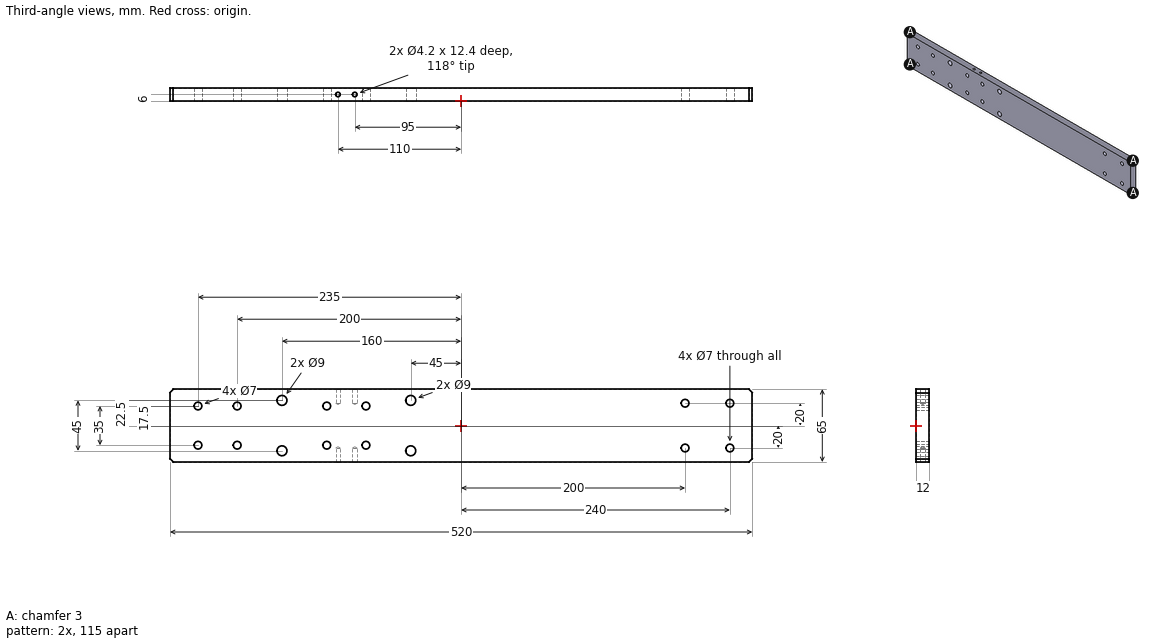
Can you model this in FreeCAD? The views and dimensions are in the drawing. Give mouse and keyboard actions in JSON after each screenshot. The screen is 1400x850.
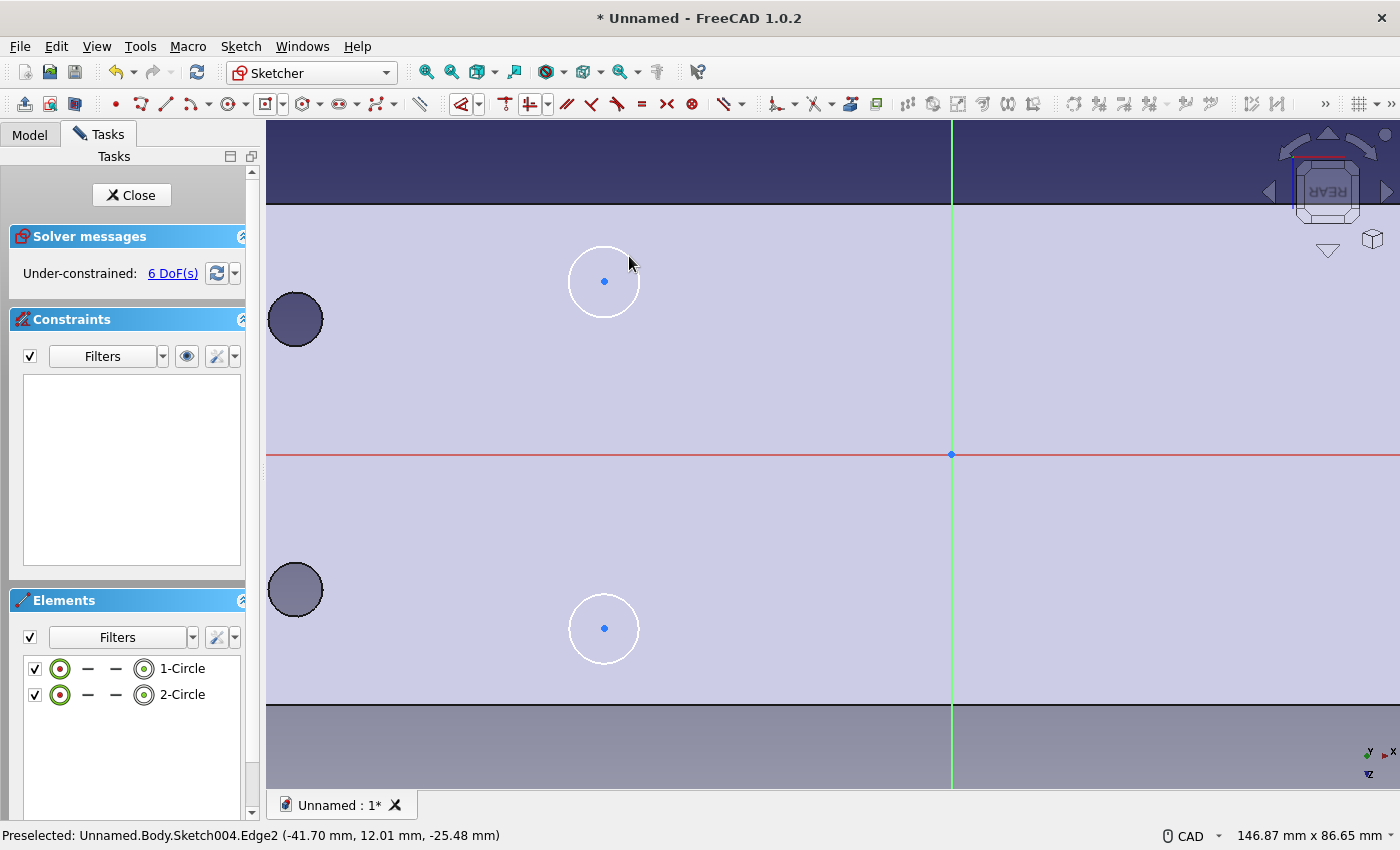
{"action": "left_click", "coordinate": [628, 604]}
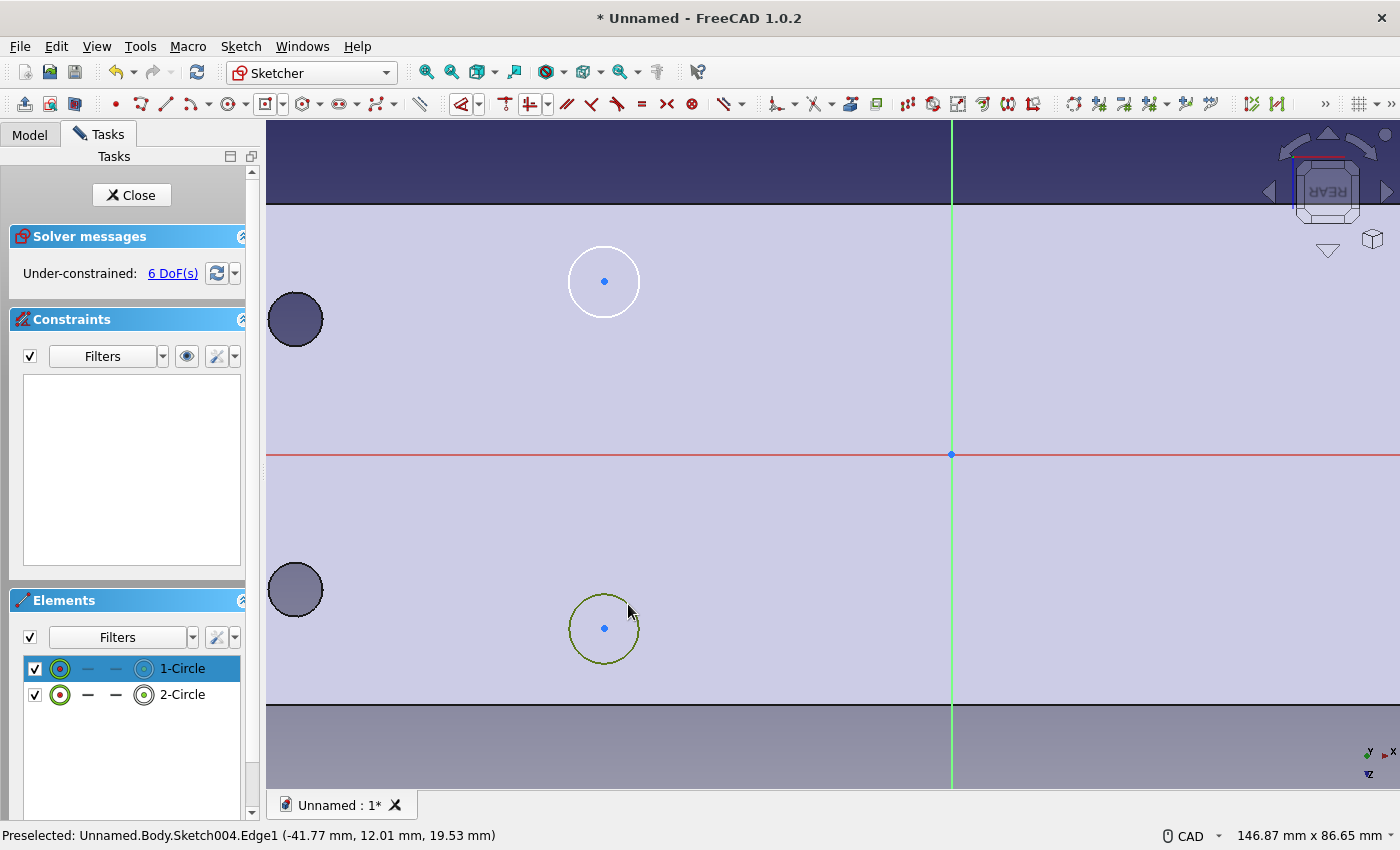
{"action": "left_click", "coordinate": [629, 257]}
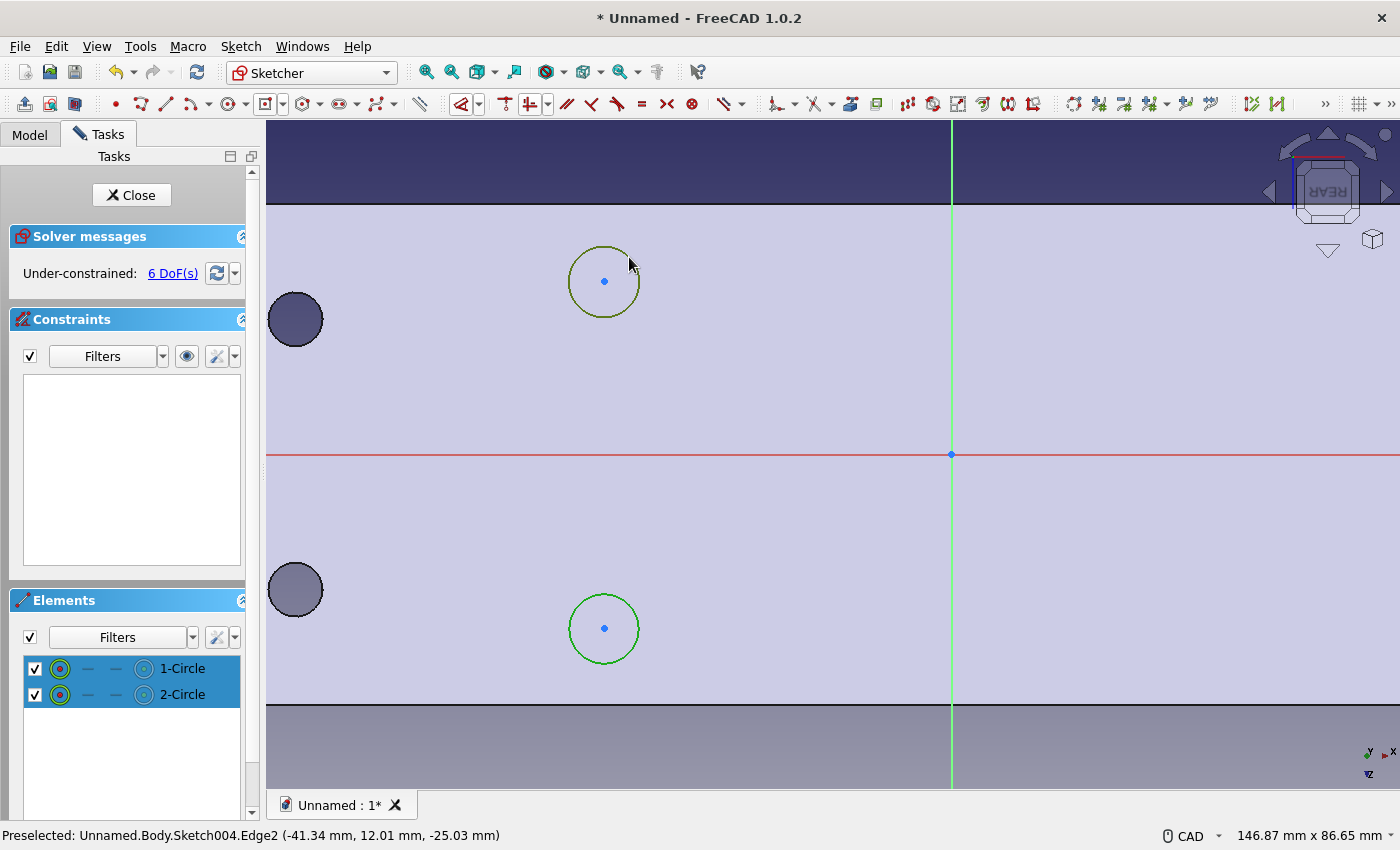
{"action": "left_click", "coordinate": [642, 104]}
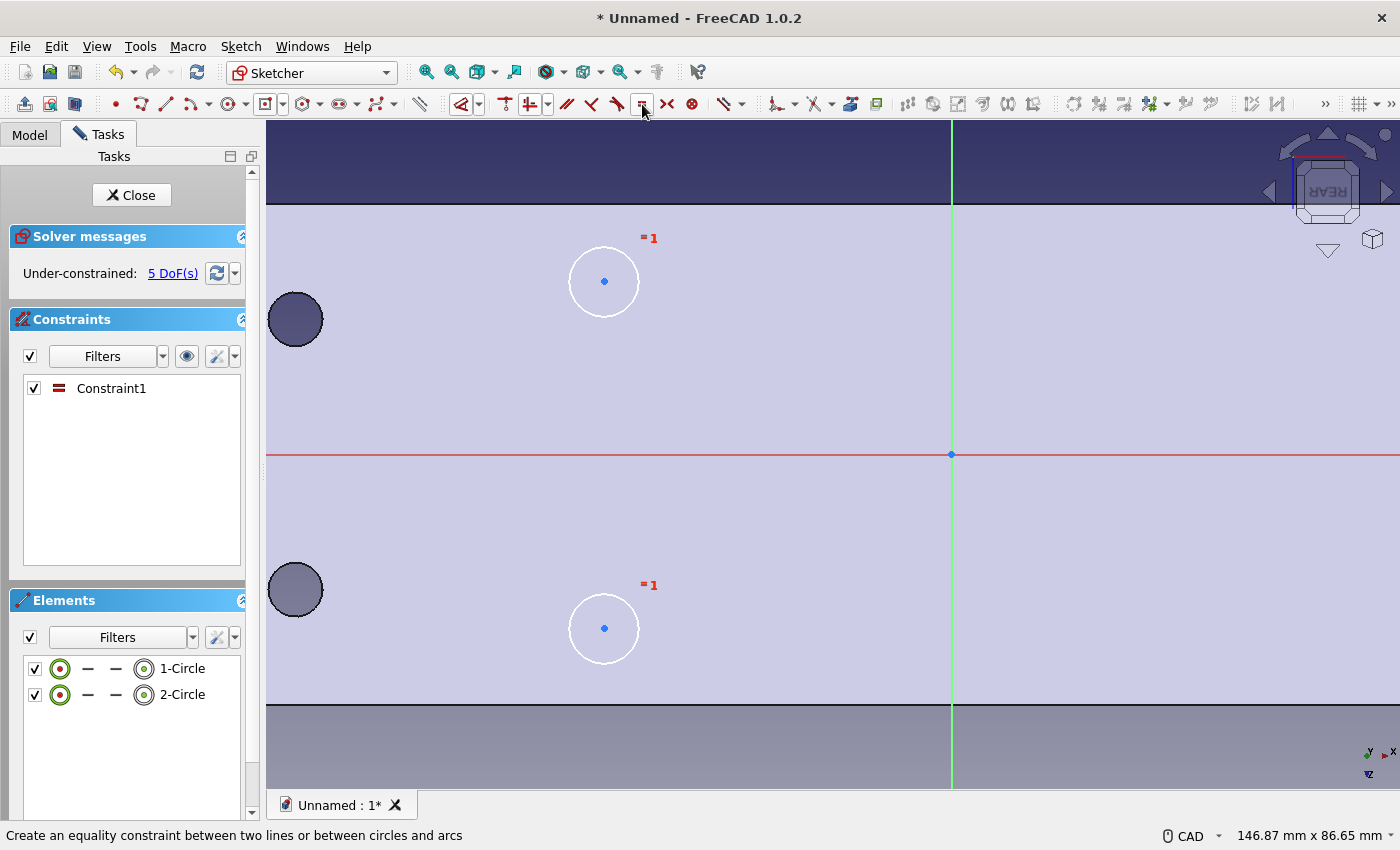
{"action": "left_click", "coordinate": [604, 629]}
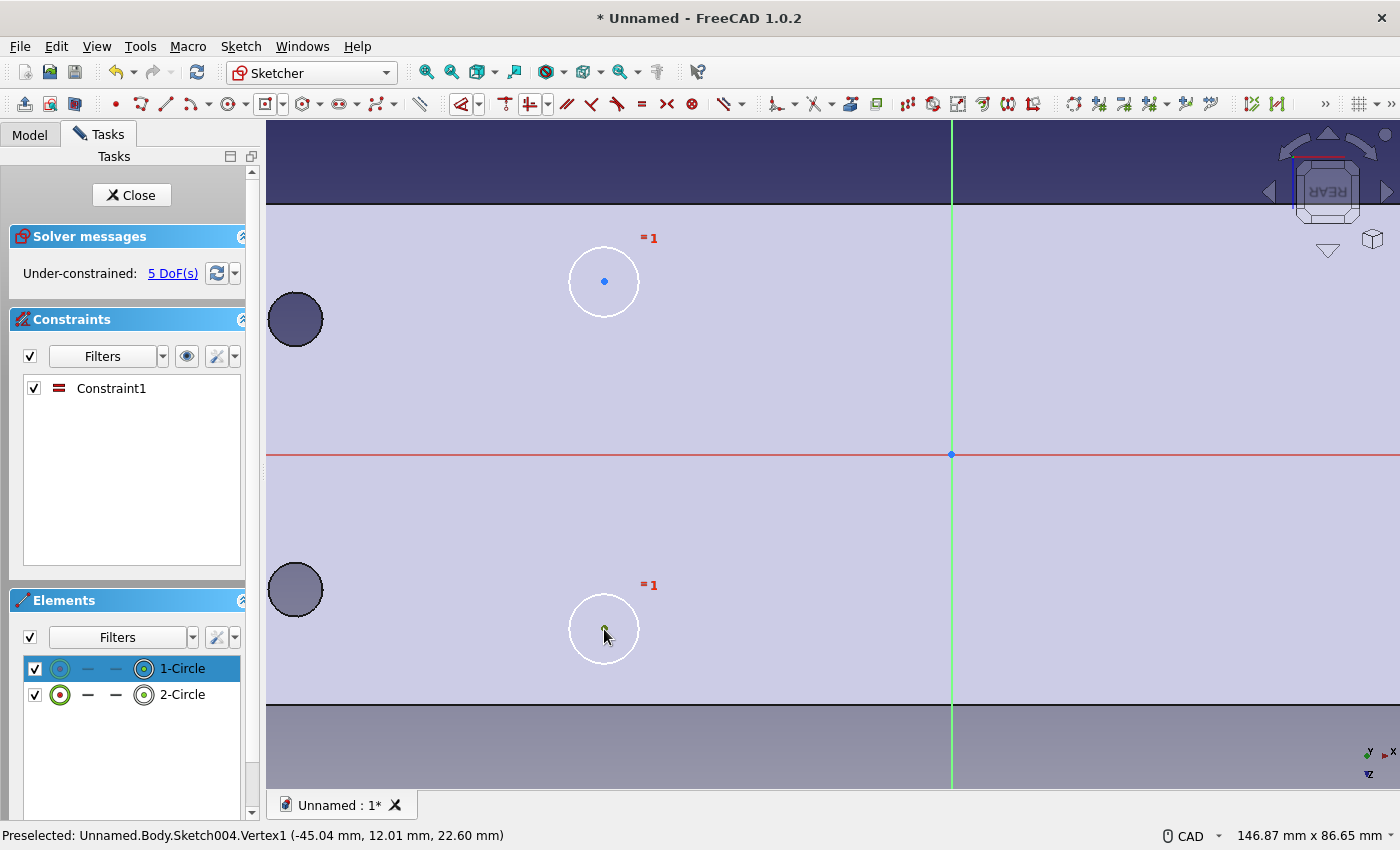
{"action": "left_click", "coordinate": [604, 282]}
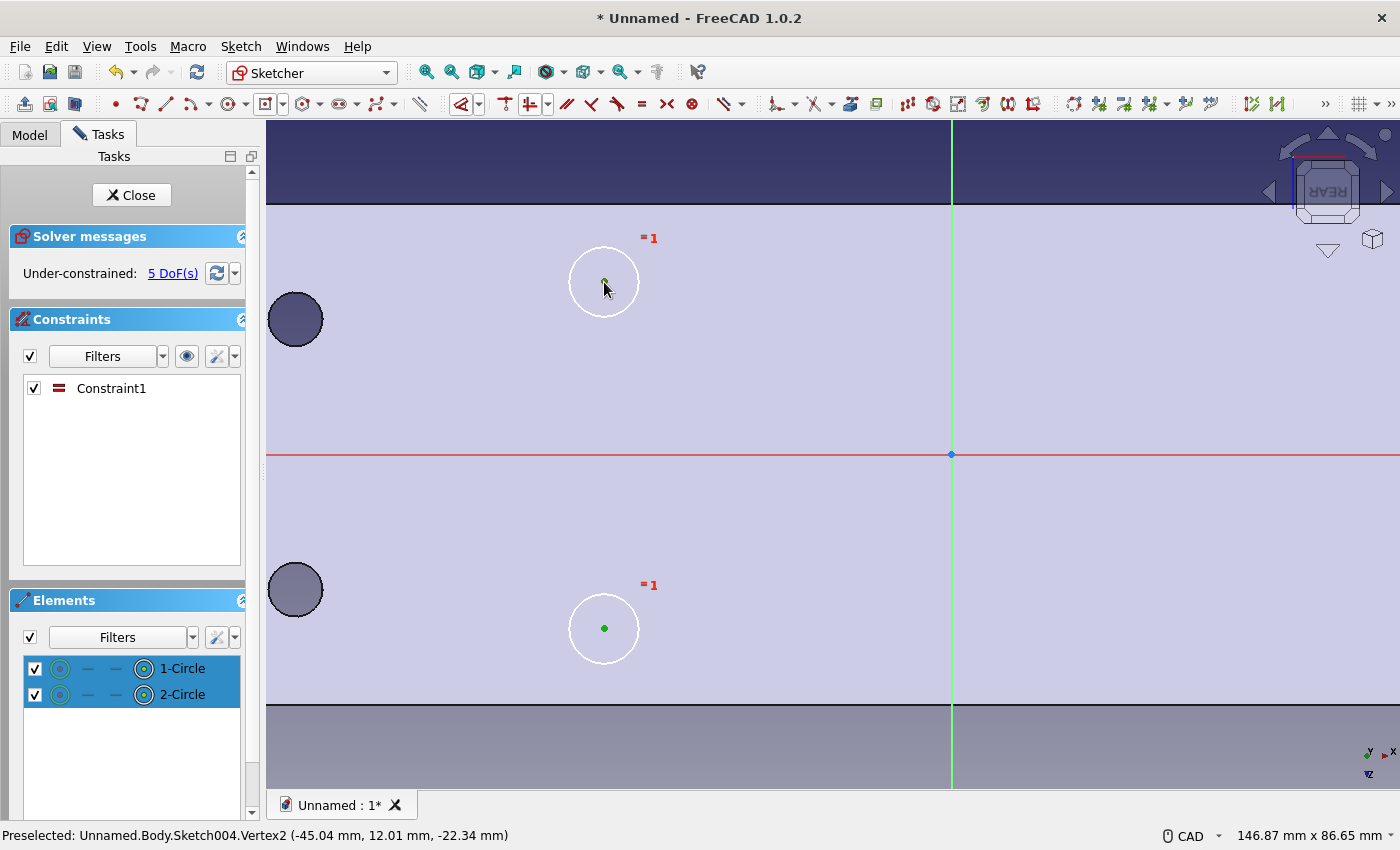
{"action": "left_click", "coordinate": [548, 104]}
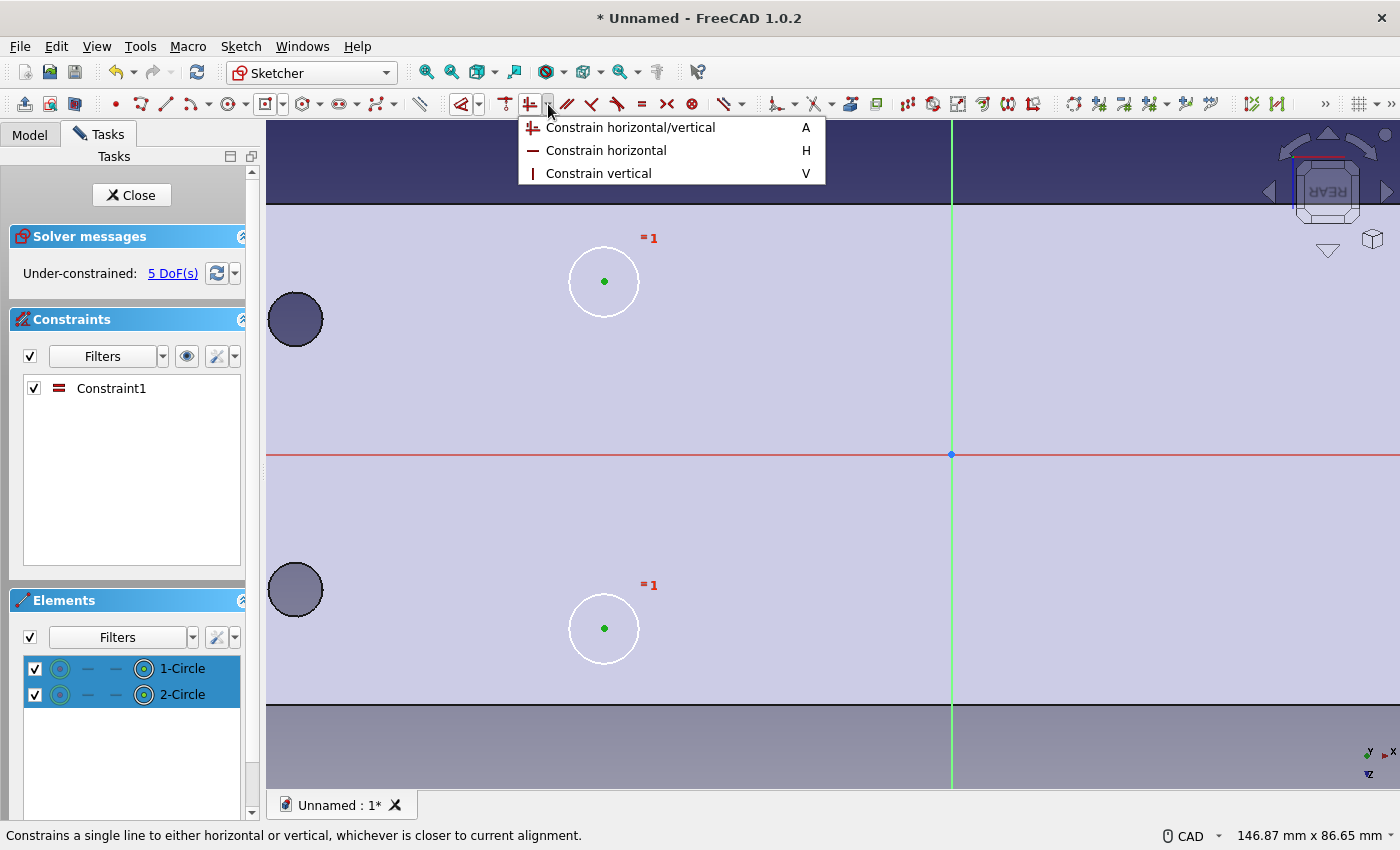
{"action": "left_click", "coordinate": [672, 174]}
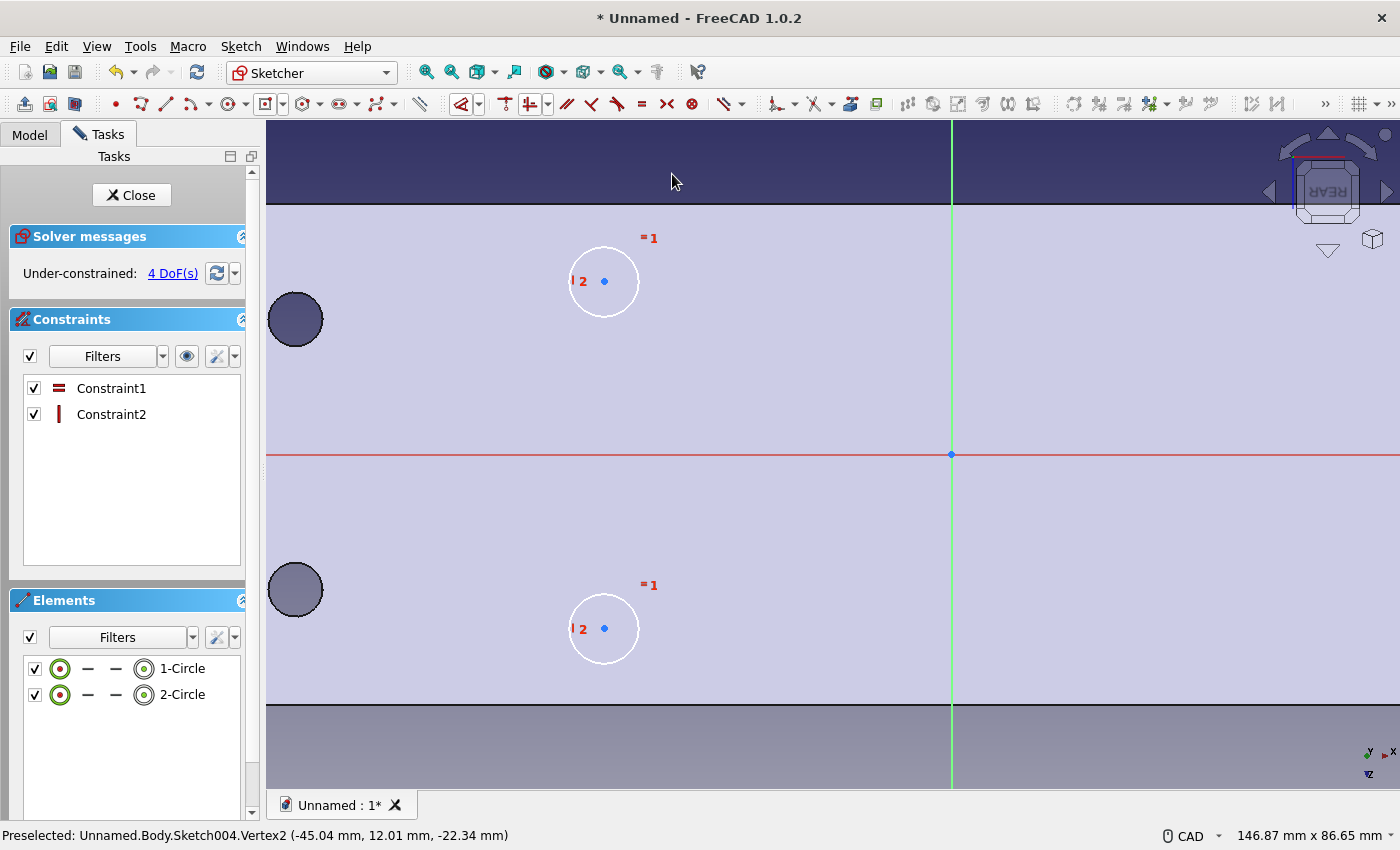
{"action": "left_click", "coordinate": [628, 604]}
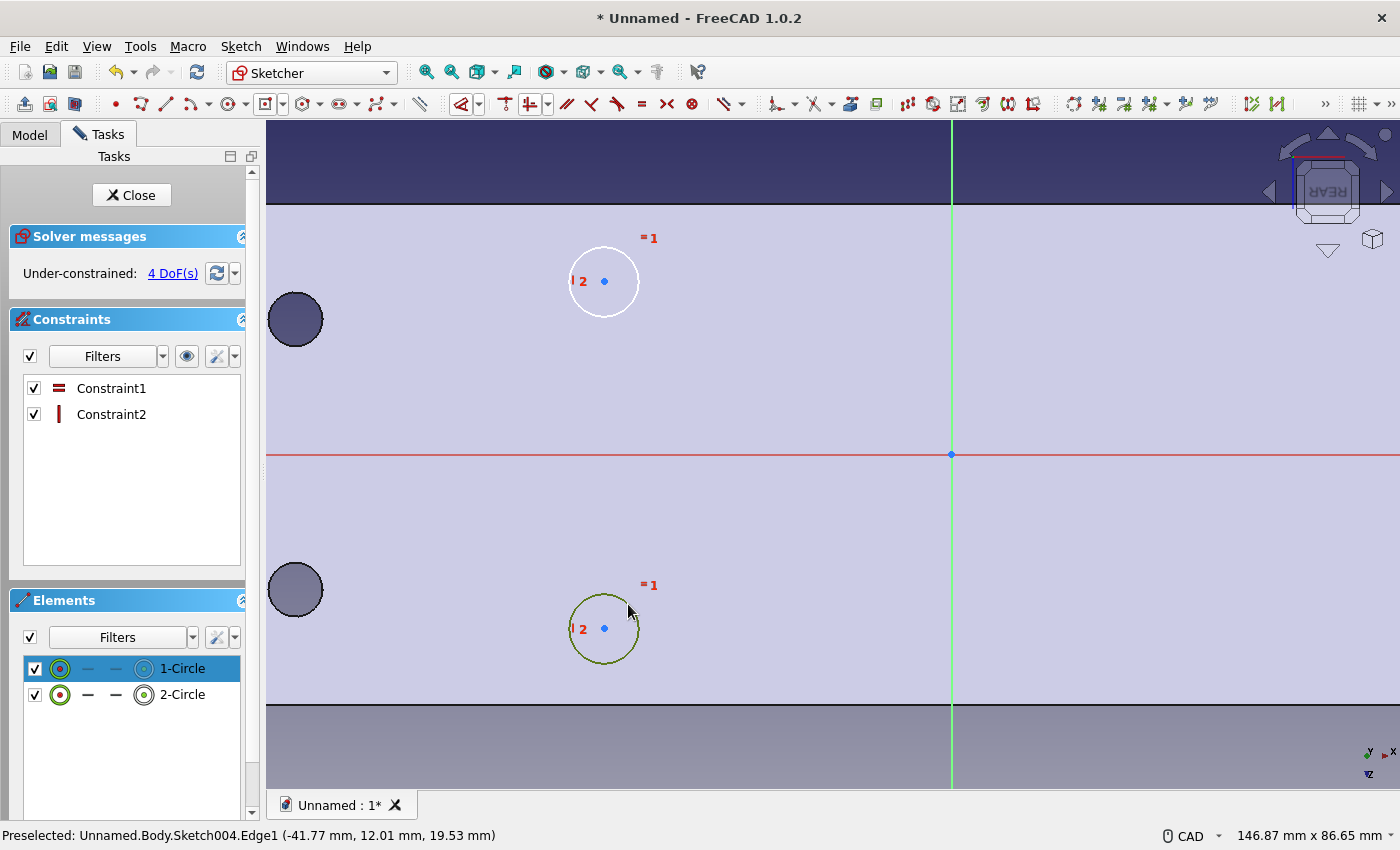
{"action": "key", "text": "k o"}